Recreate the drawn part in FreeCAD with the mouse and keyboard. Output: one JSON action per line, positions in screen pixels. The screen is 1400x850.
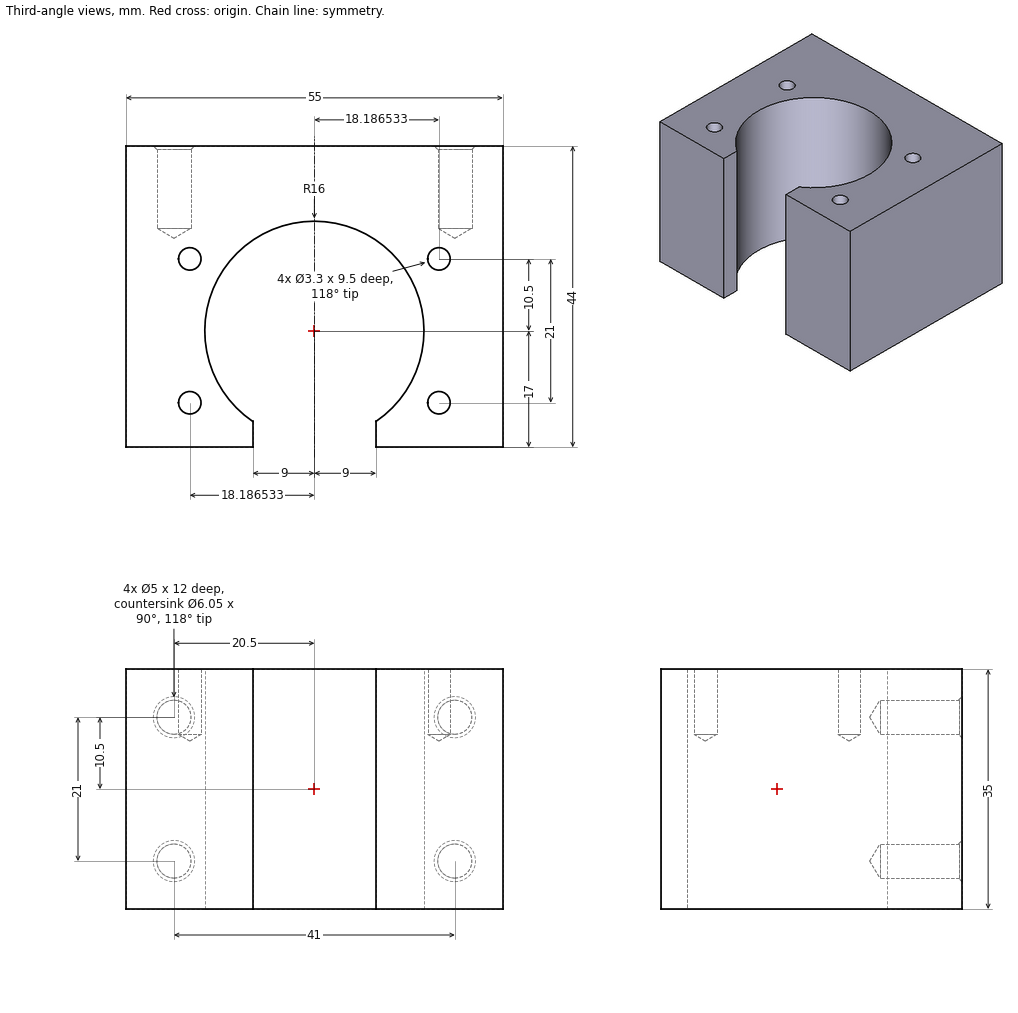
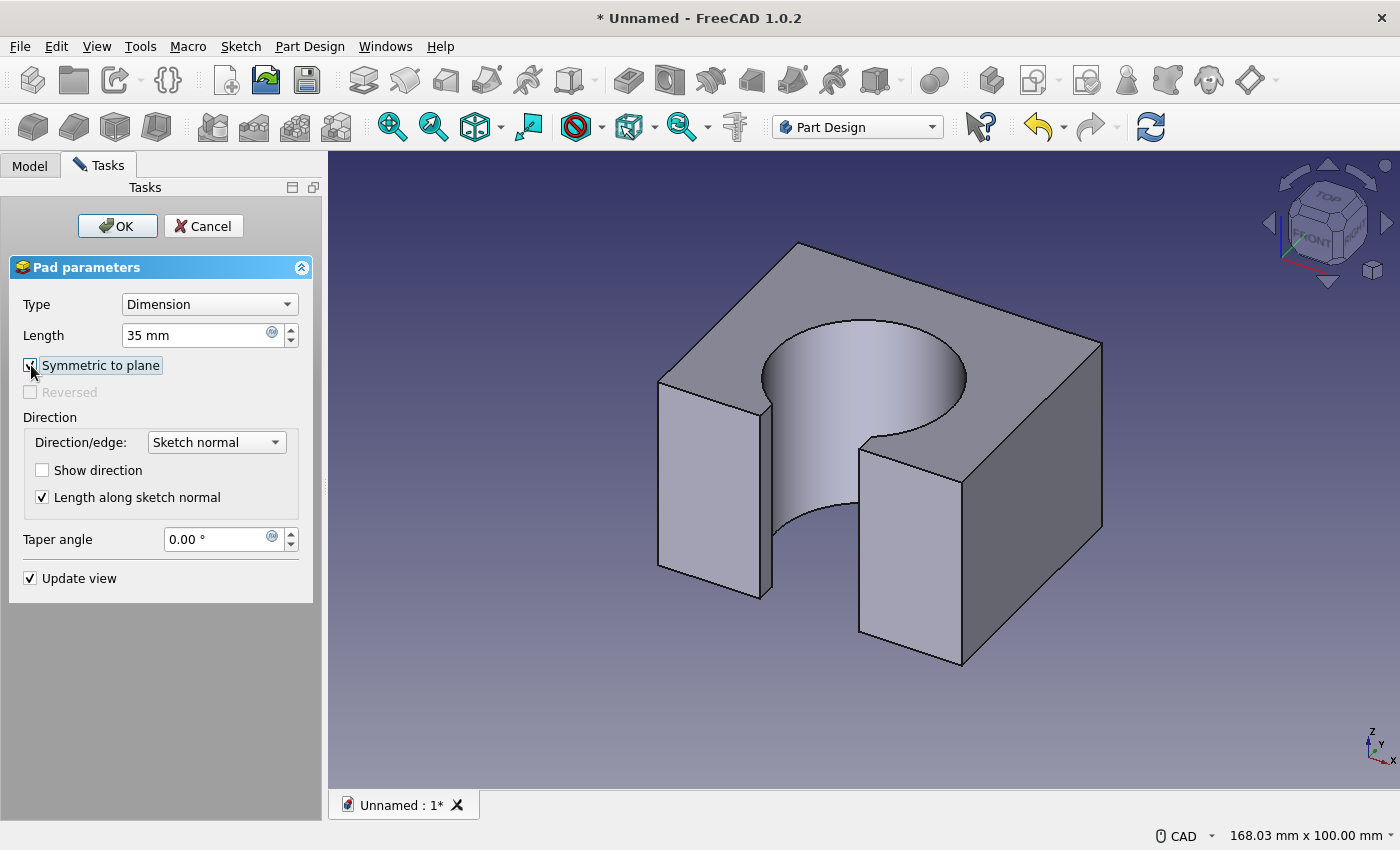
{"action": "left_click", "coordinate": [118, 226]}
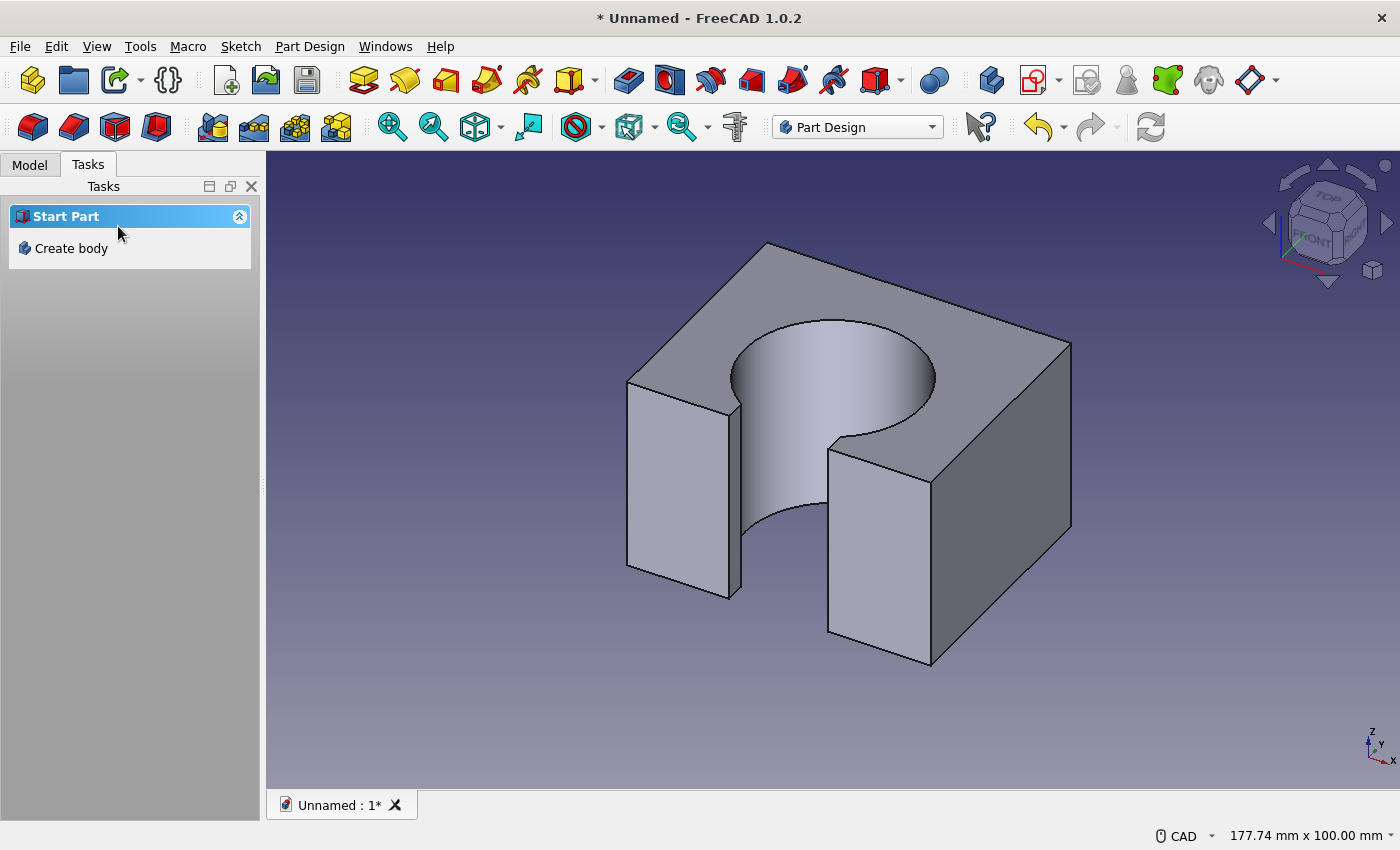
{"action": "left_click", "coordinate": [976, 351]}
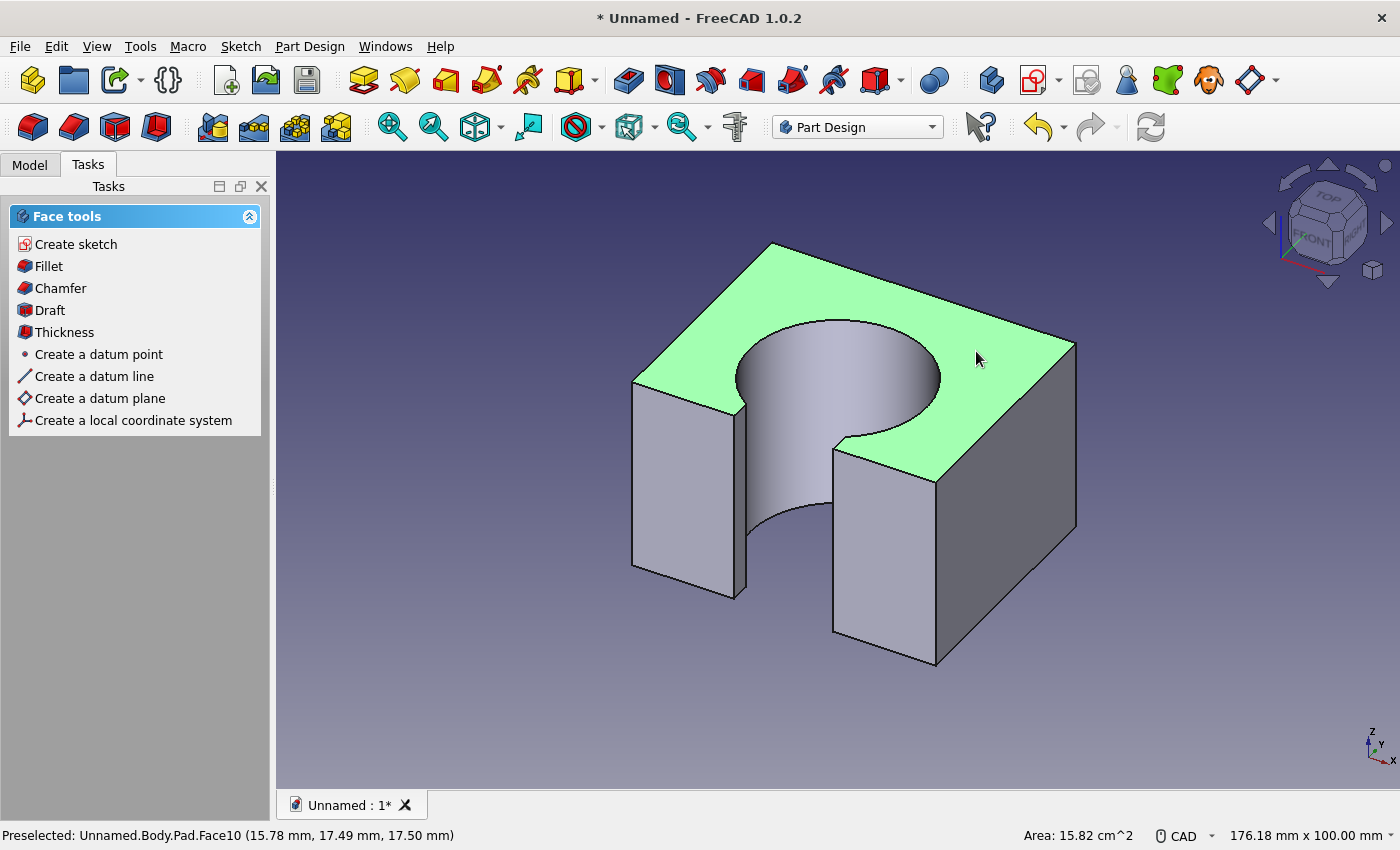
{"action": "left_click", "coordinate": [1032, 80]}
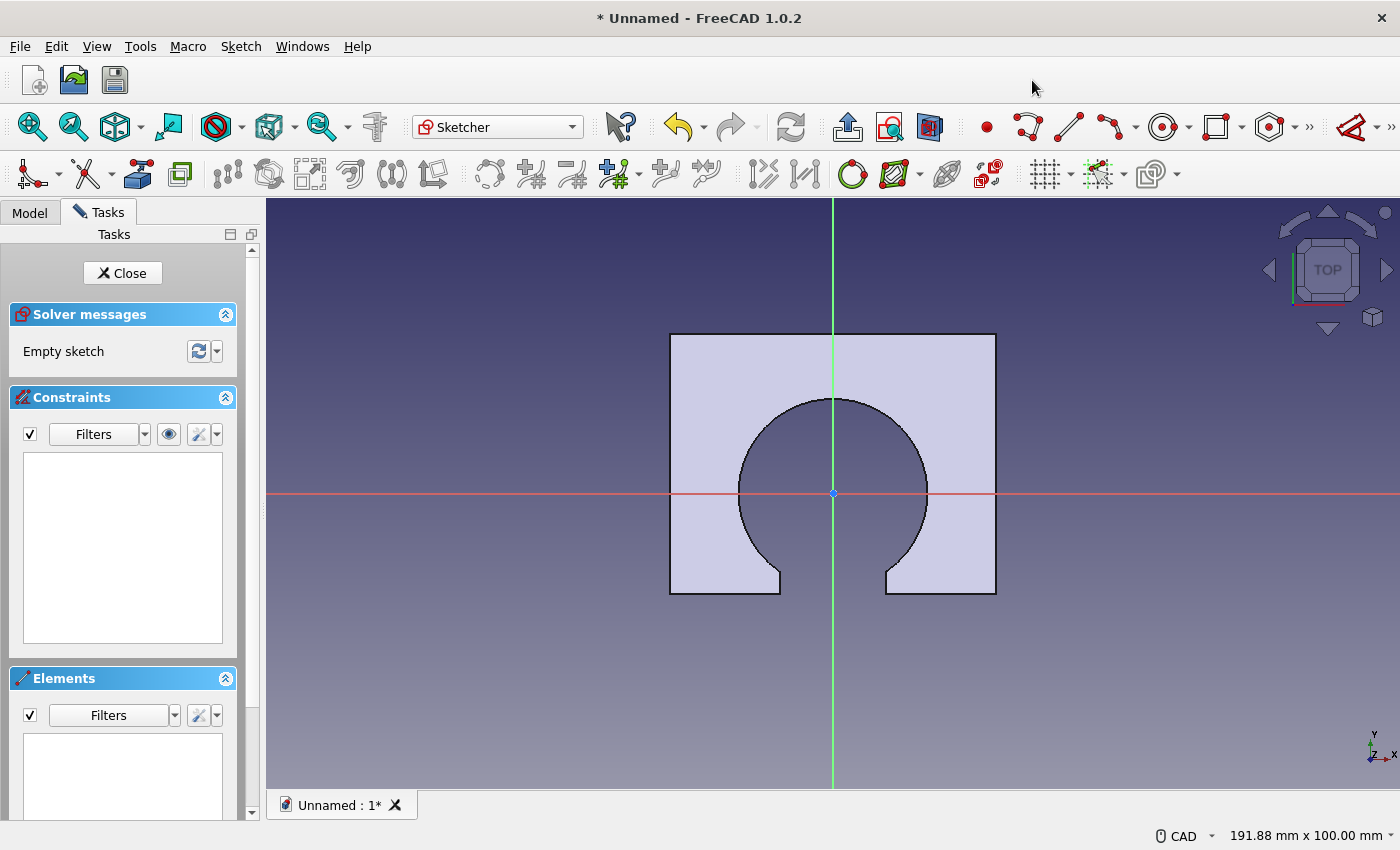
{"action": "scroll", "coordinate": [873, 493], "scroll_direction": "up", "scroll_amount": 5}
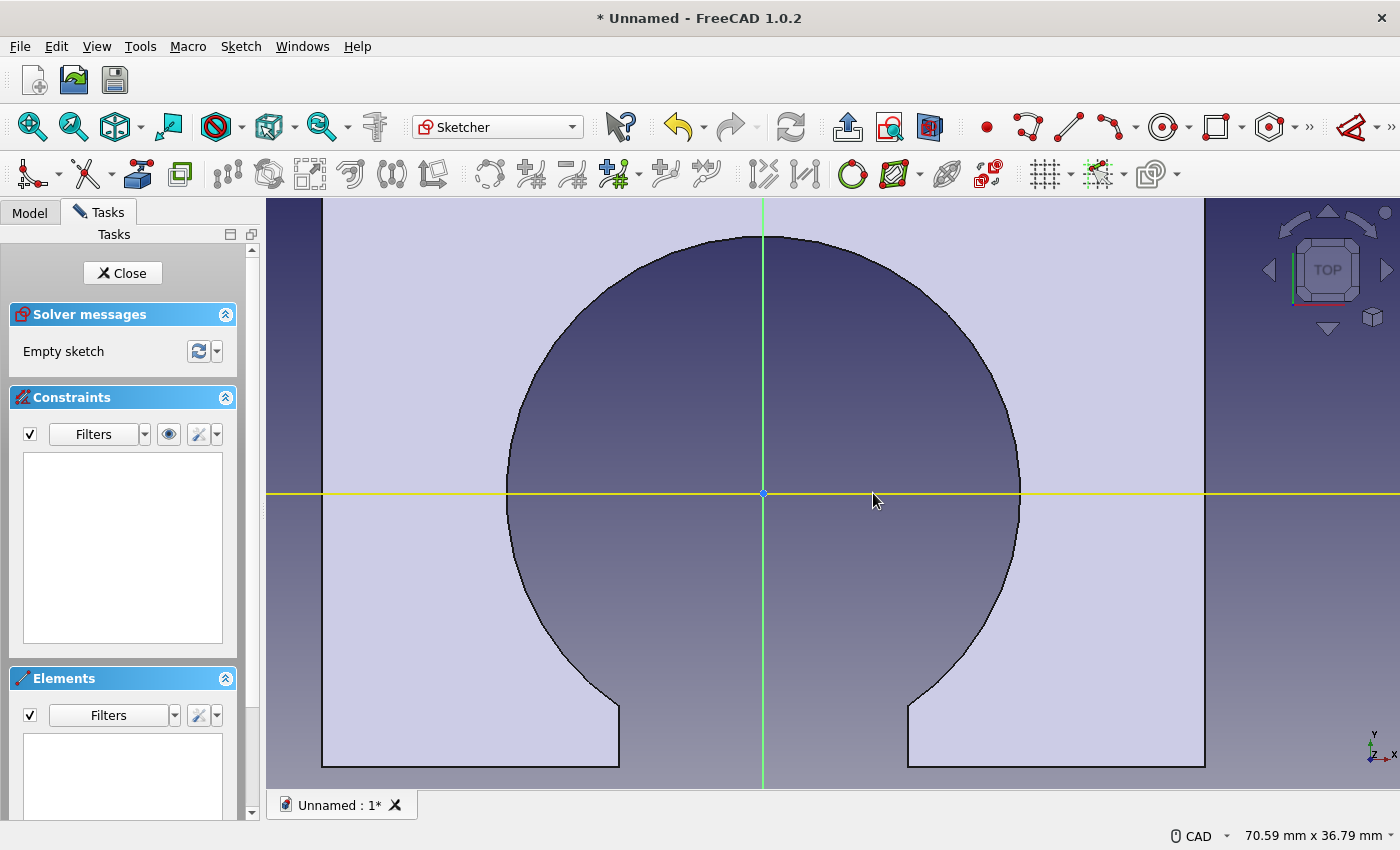
{"action": "left_click", "coordinate": [1162, 128]}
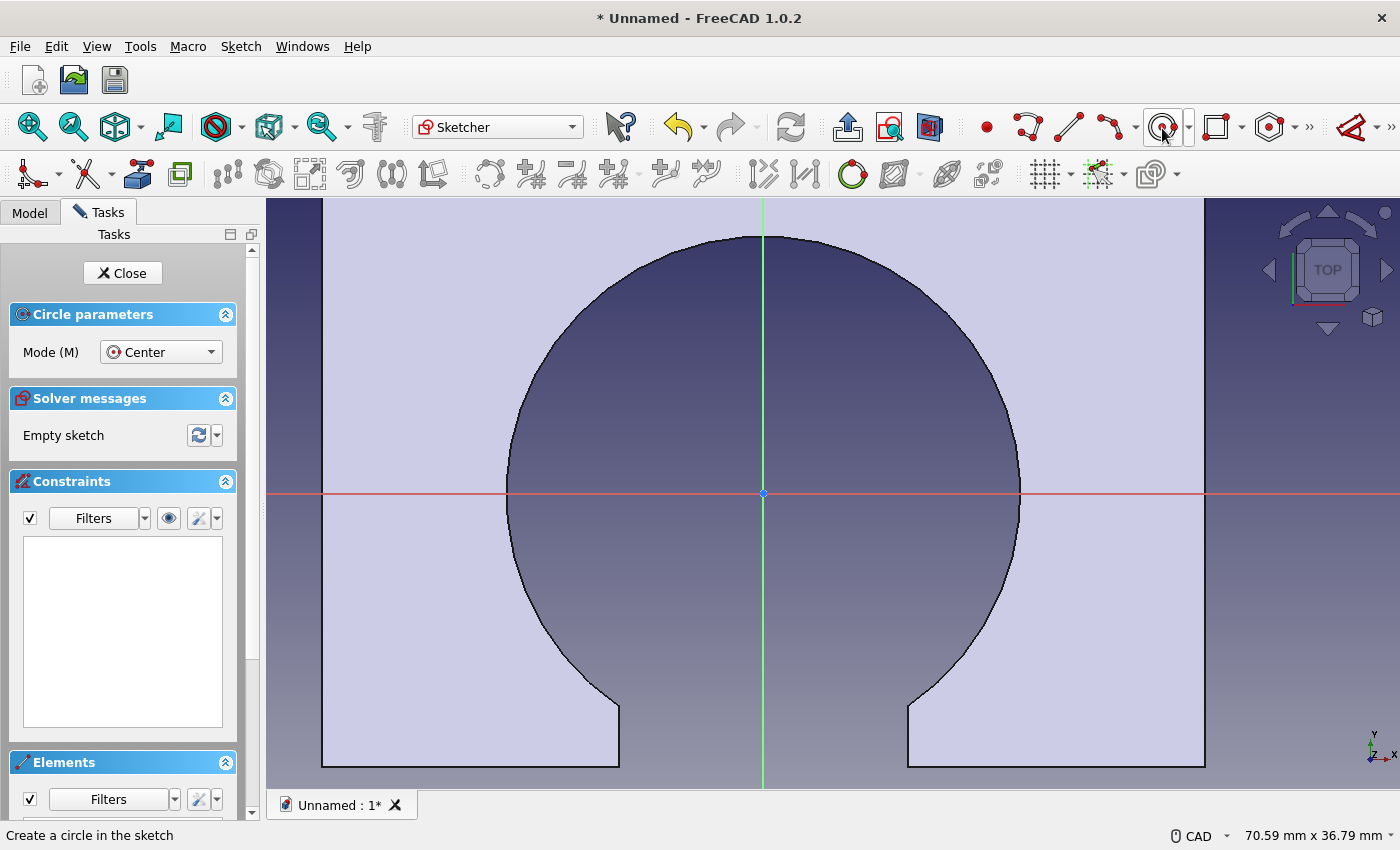
{"action": "left_click", "coordinate": [1056, 325]}
{"action": "mouse_move", "coordinate": [1074, 306]}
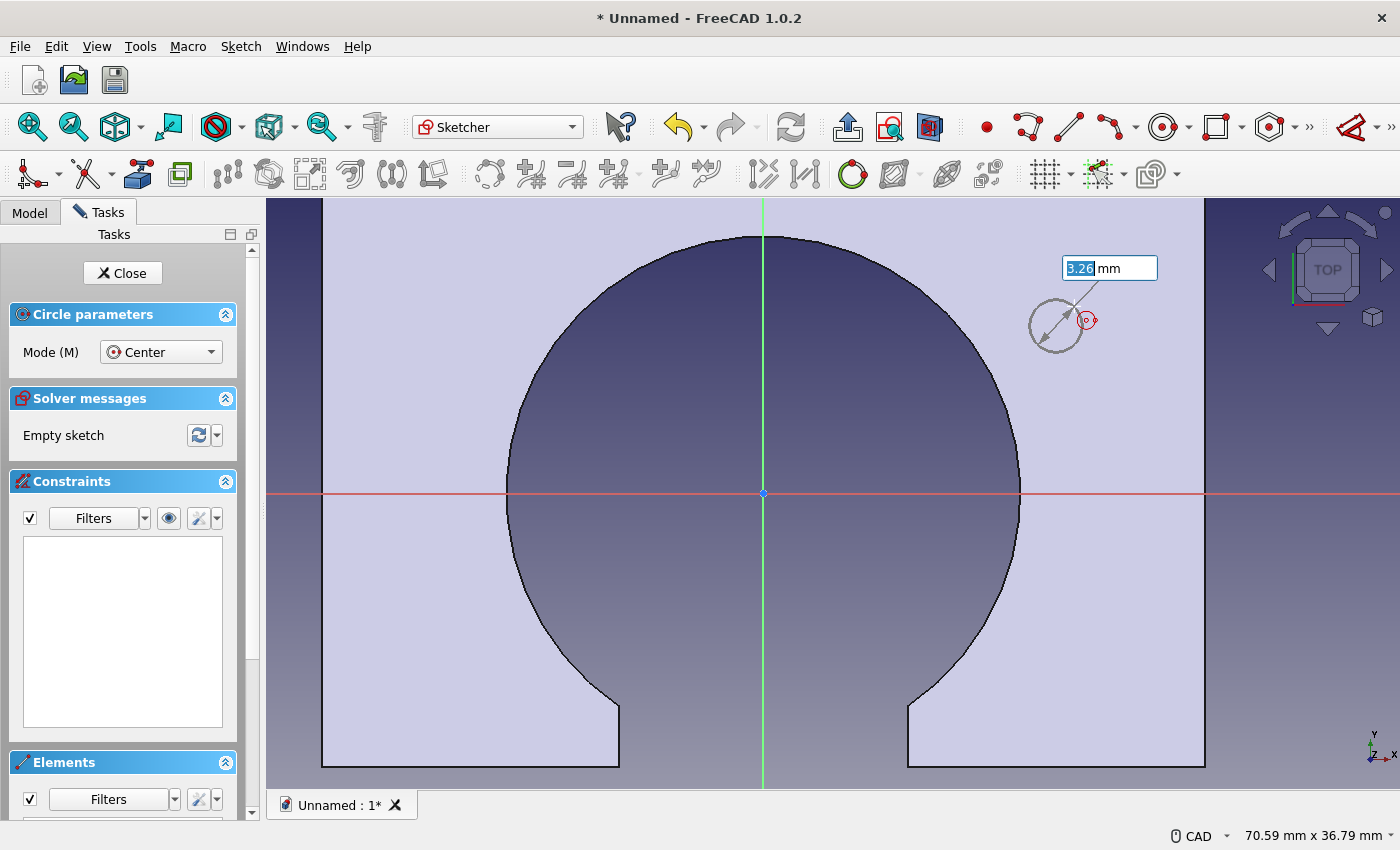
{"action": "type", "text": "3.3"}
{"action": "key", "text": "Return"}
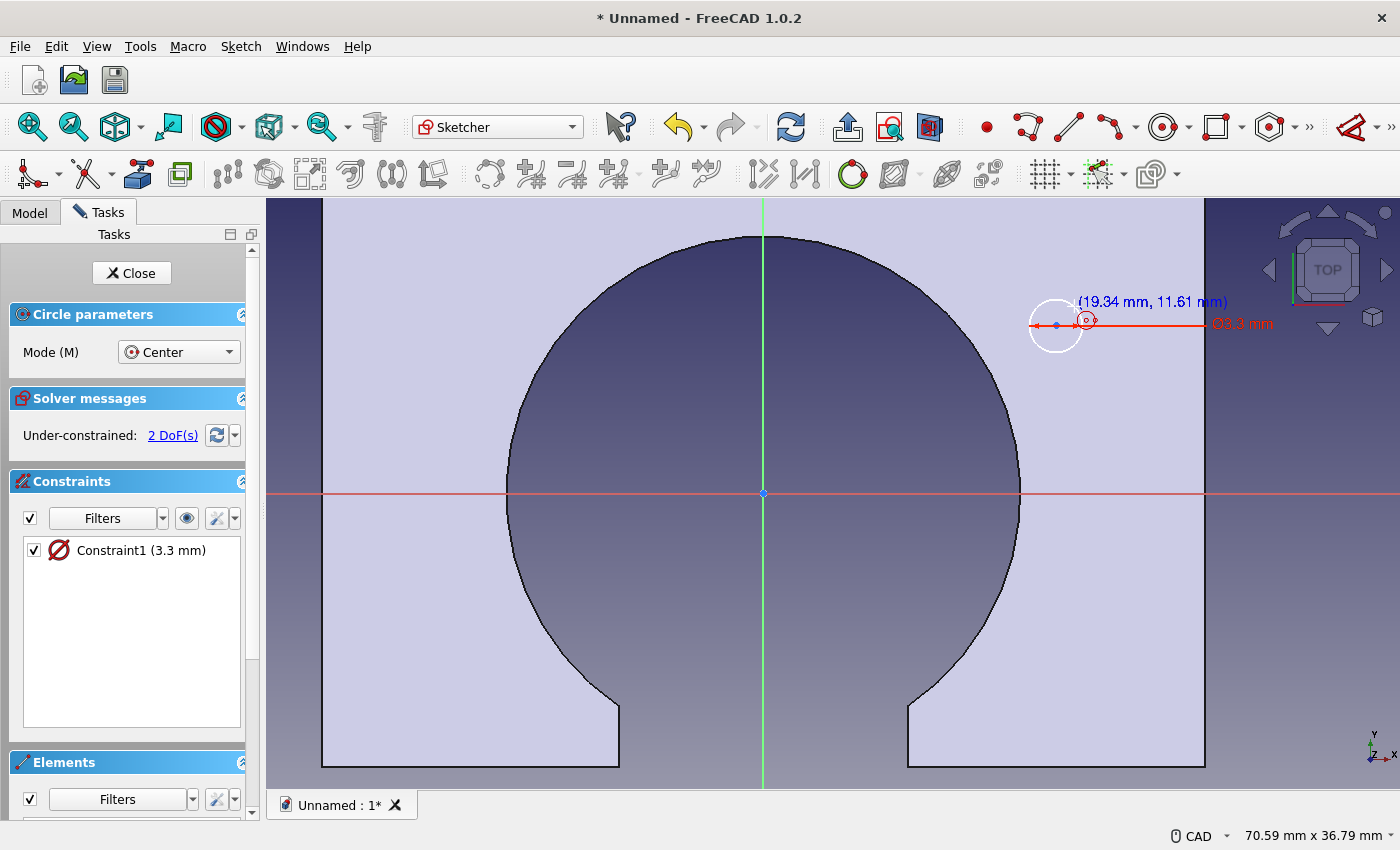
{"action": "left_click", "coordinate": [1056, 662]}
{"action": "mouse_move", "coordinate": [1074, 643]}